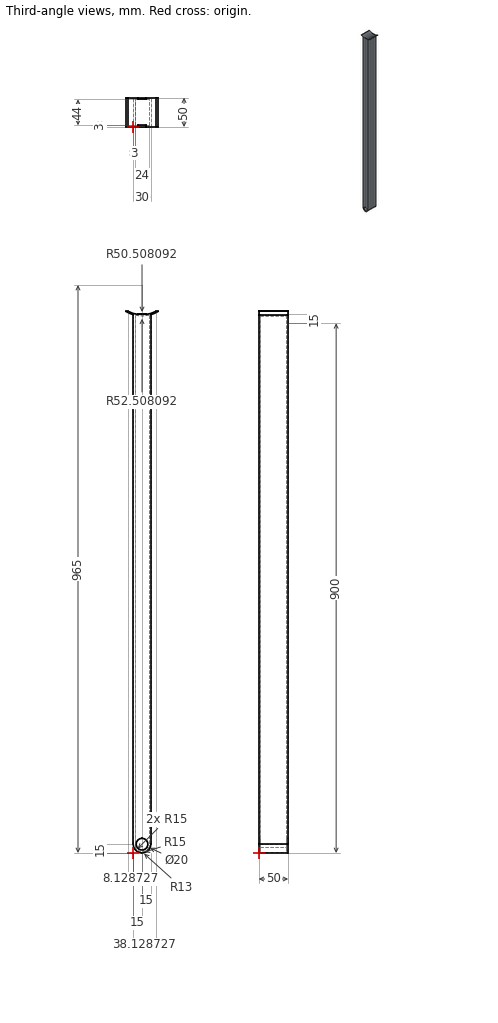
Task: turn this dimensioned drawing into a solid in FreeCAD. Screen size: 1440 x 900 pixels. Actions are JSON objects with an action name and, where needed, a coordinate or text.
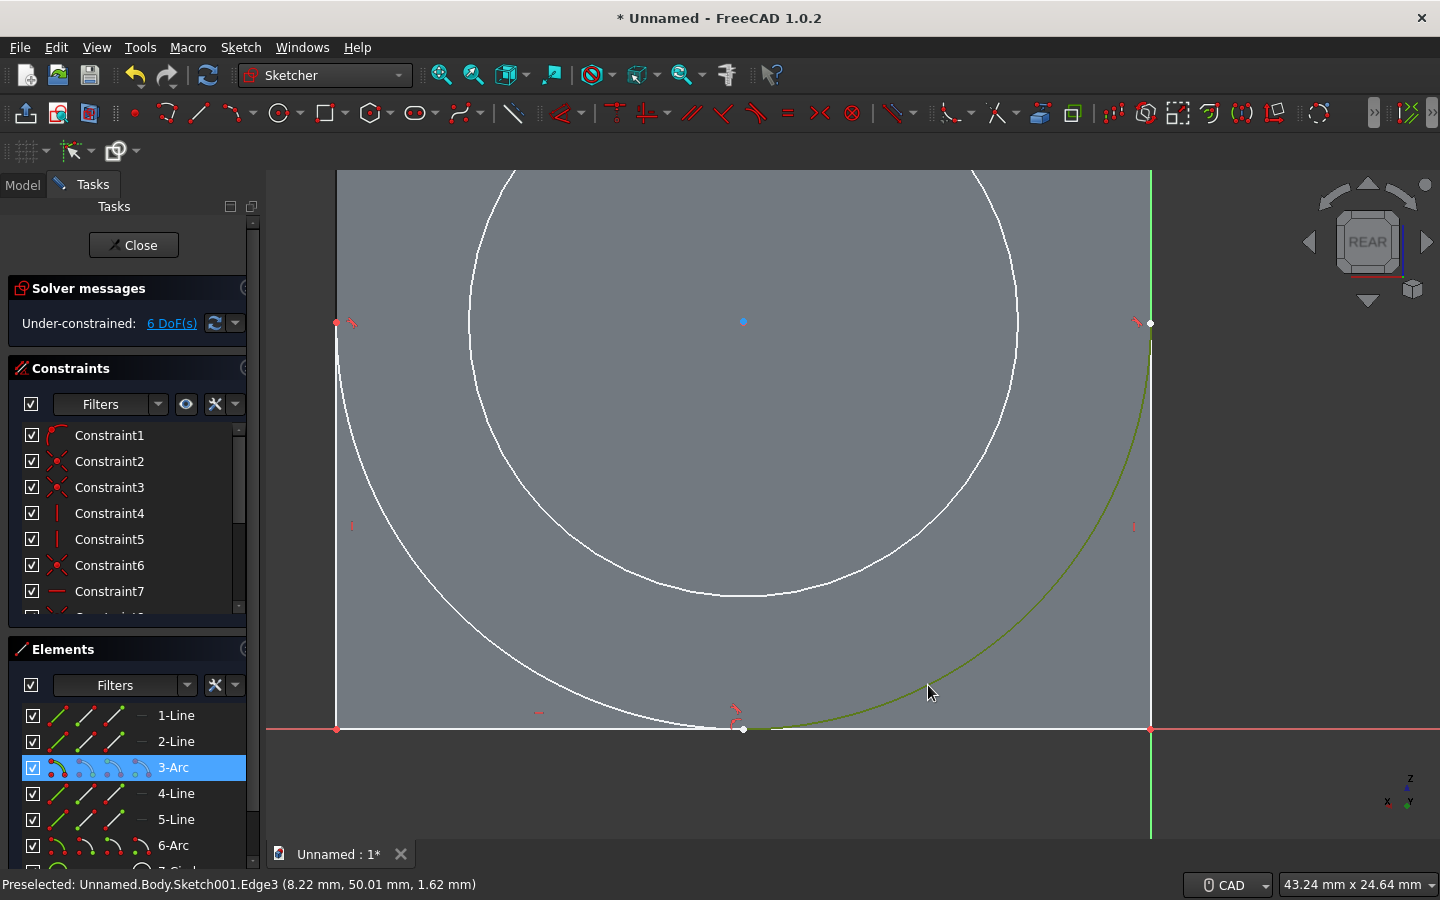
{"action": "left_click", "coordinate": [381, 507]}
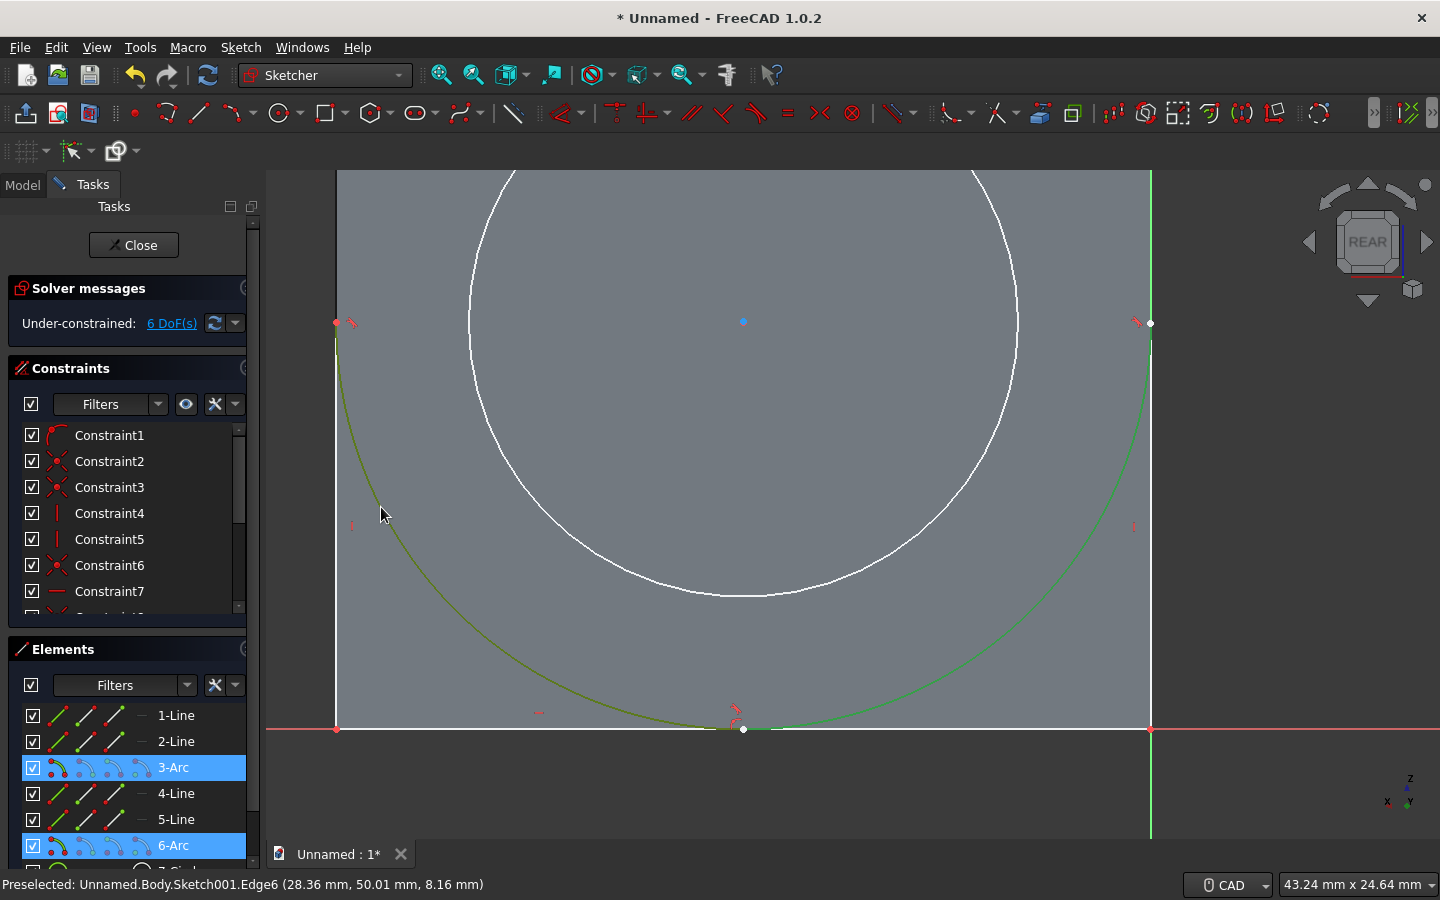
{"action": "left_click", "coordinate": [788, 114]}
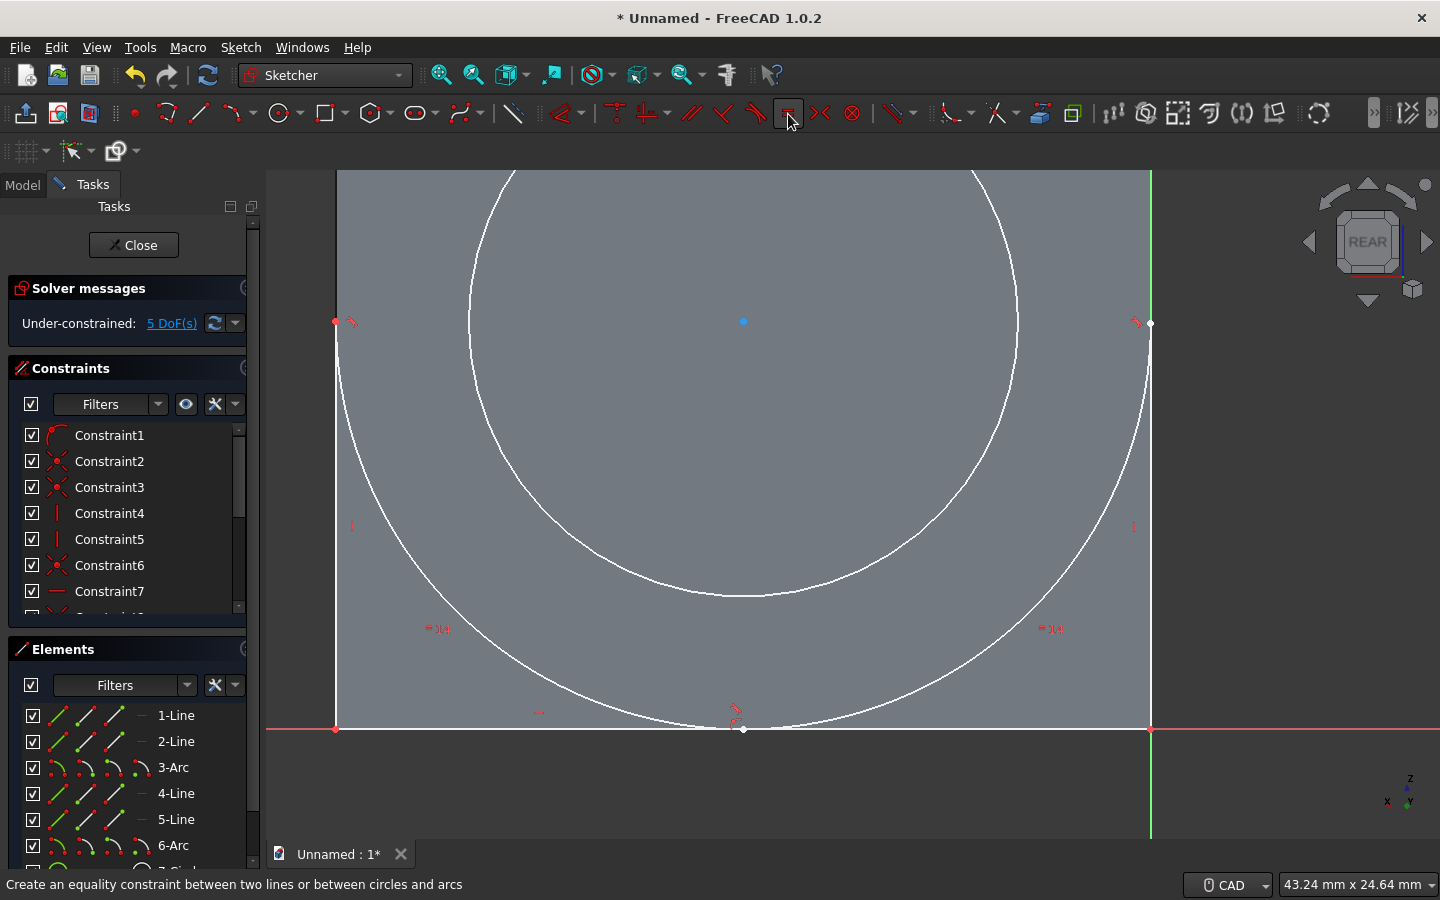
{"action": "left_click", "coordinate": [560, 114]}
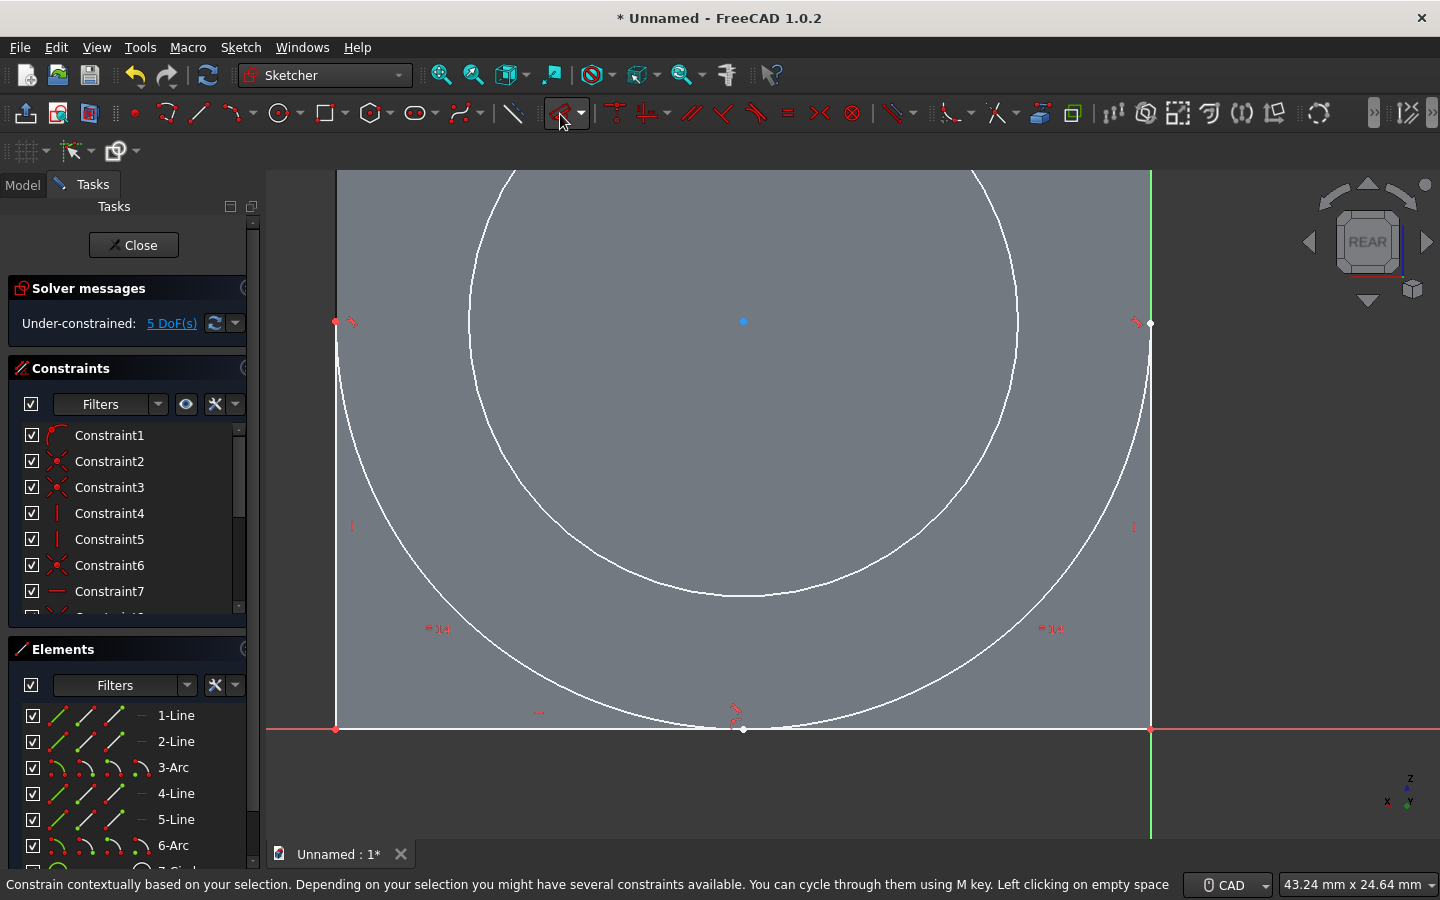
{"action": "left_click", "coordinate": [928, 685]}
{"action": "left_click", "coordinate": [943, 714]}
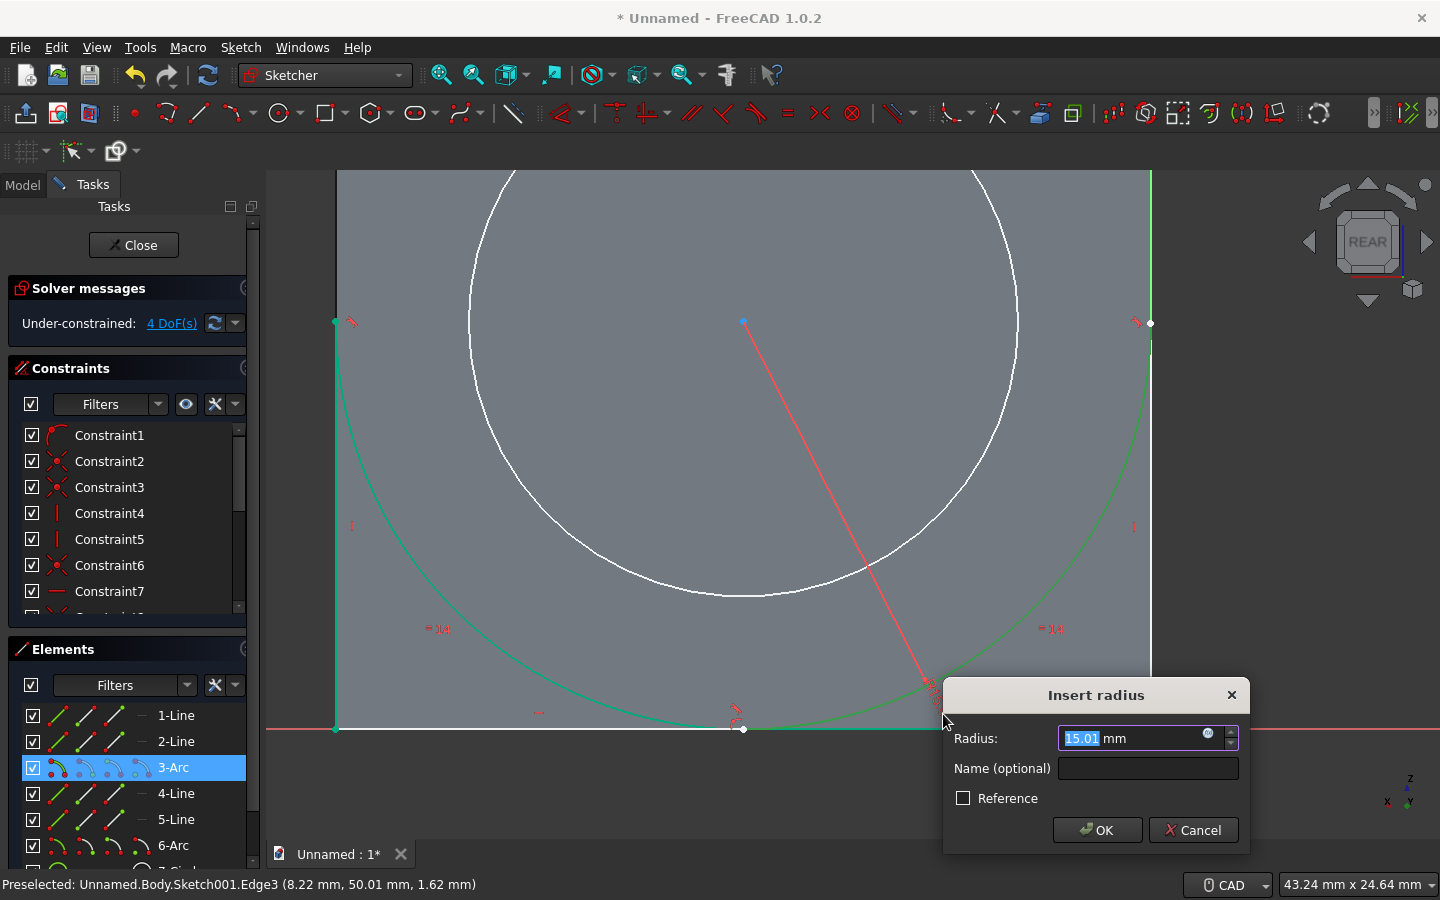
{"action": "type", "text": "15"}
{"action": "key", "text": "Return"}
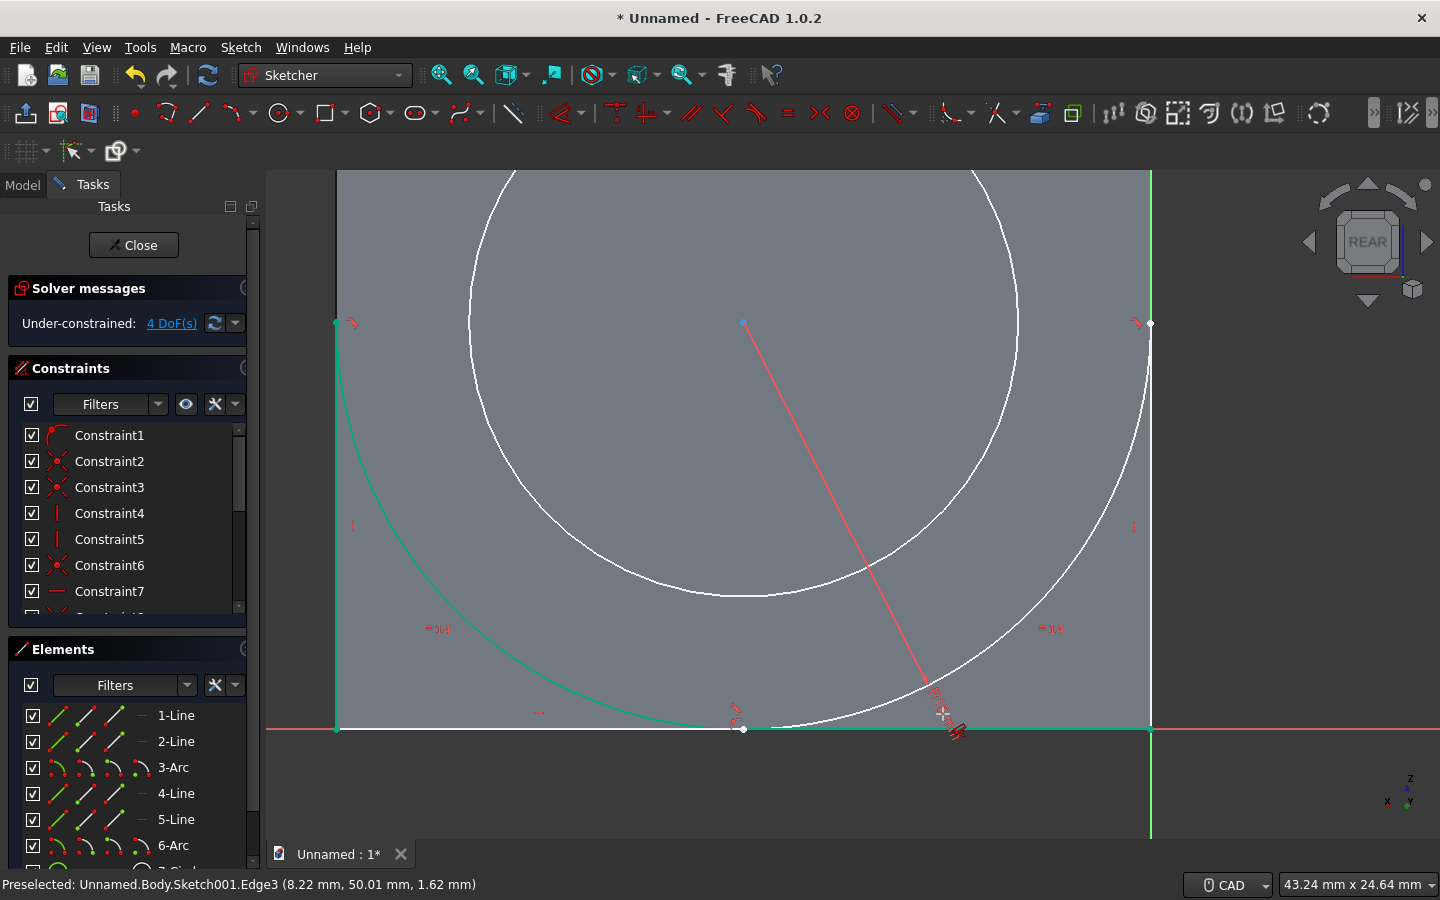
{"action": "left_click", "coordinate": [550, 517]}
{"action": "left_click", "coordinate": [527, 540]}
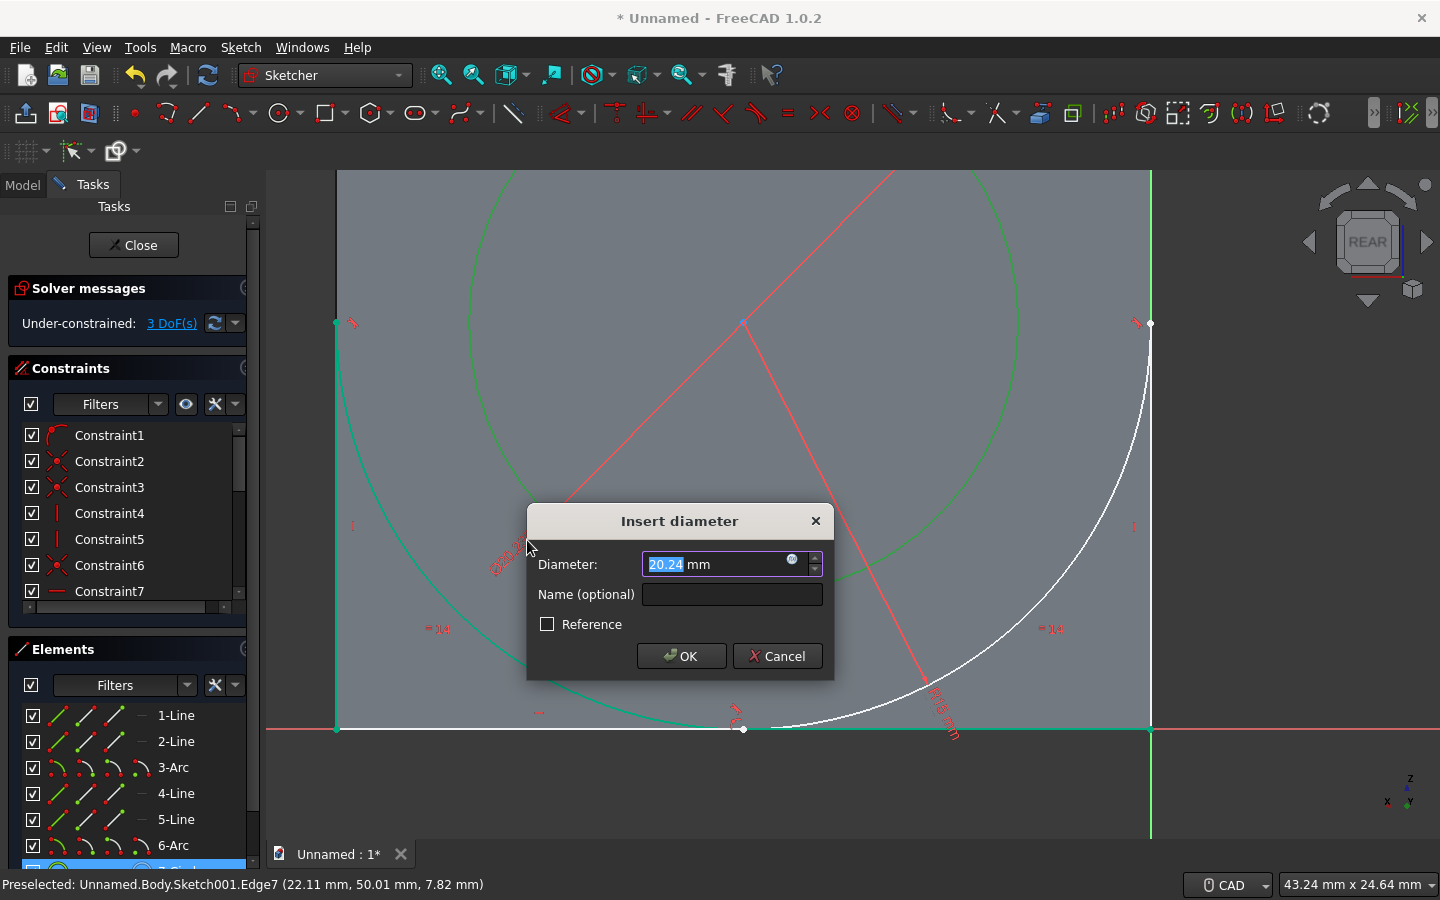
{"action": "type", "text": "20"}
{"action": "key", "text": "Return"}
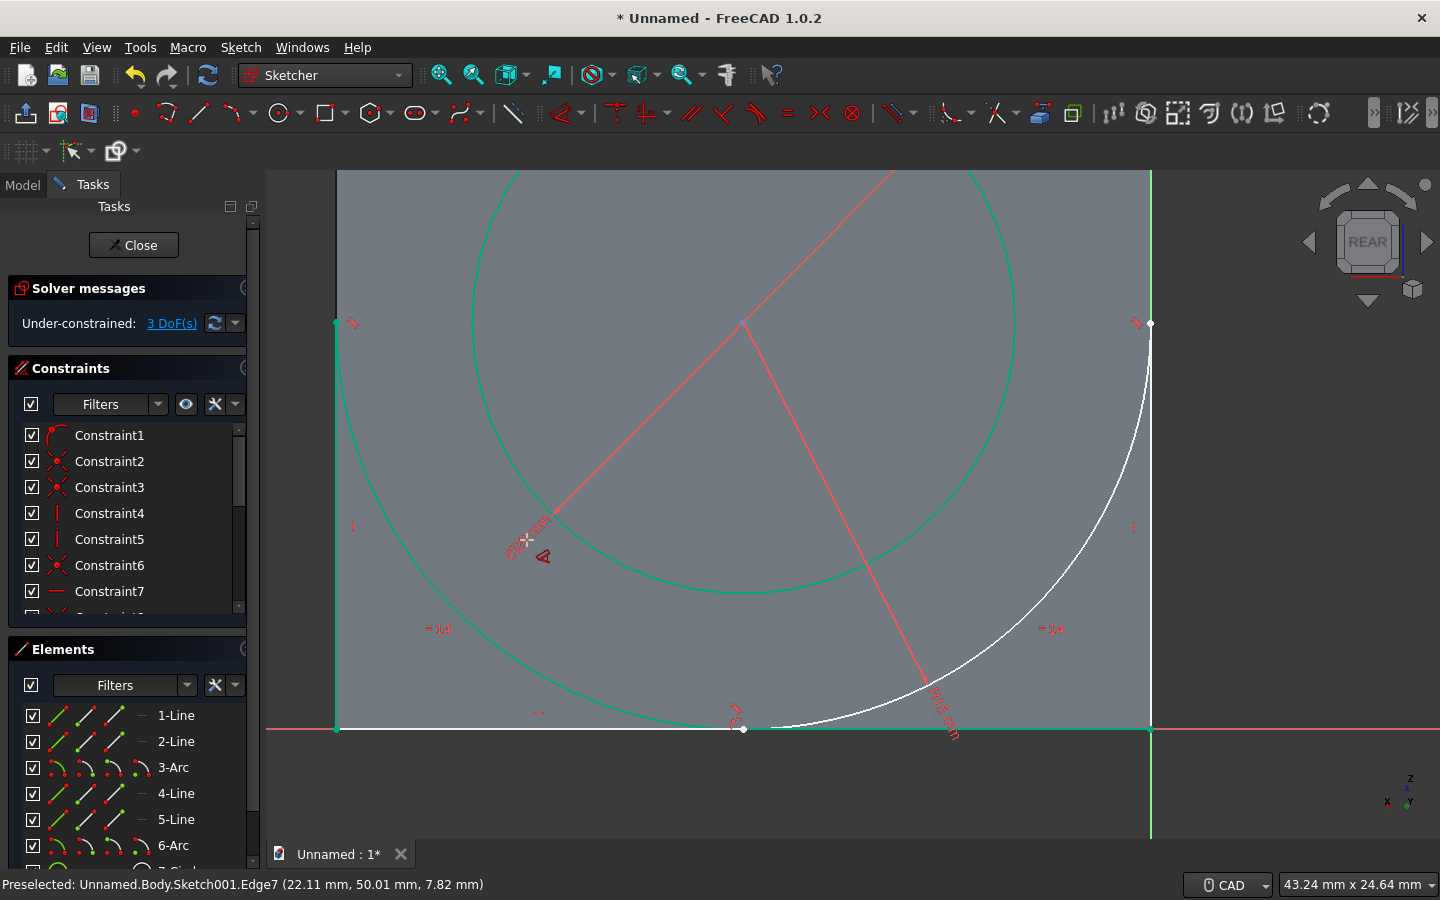
{"action": "left_click", "coordinate": [1151, 608]}
{"action": "left_click", "coordinate": [1185, 527]}